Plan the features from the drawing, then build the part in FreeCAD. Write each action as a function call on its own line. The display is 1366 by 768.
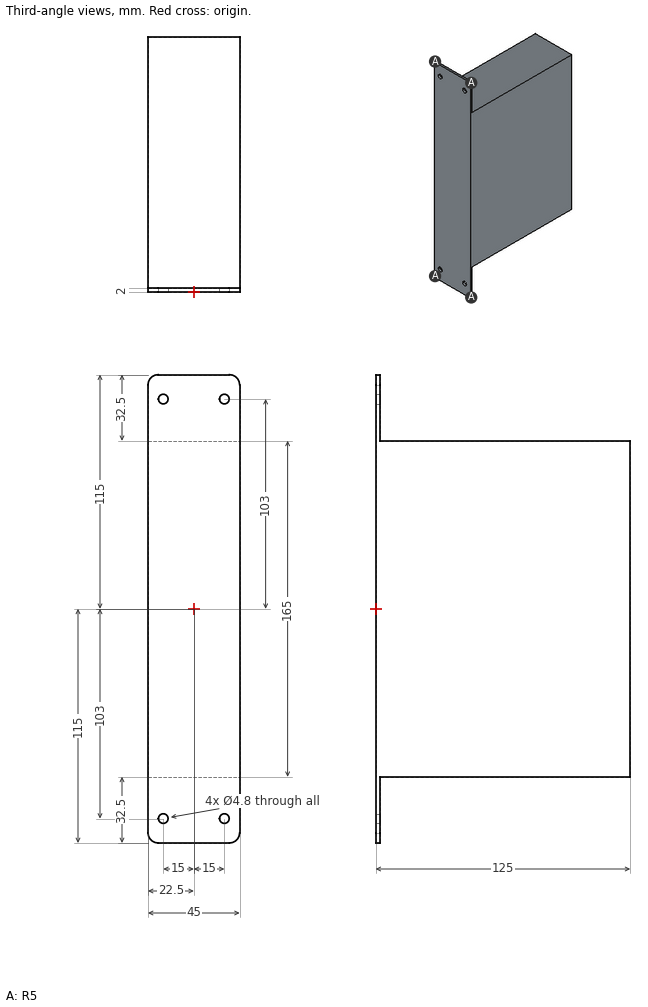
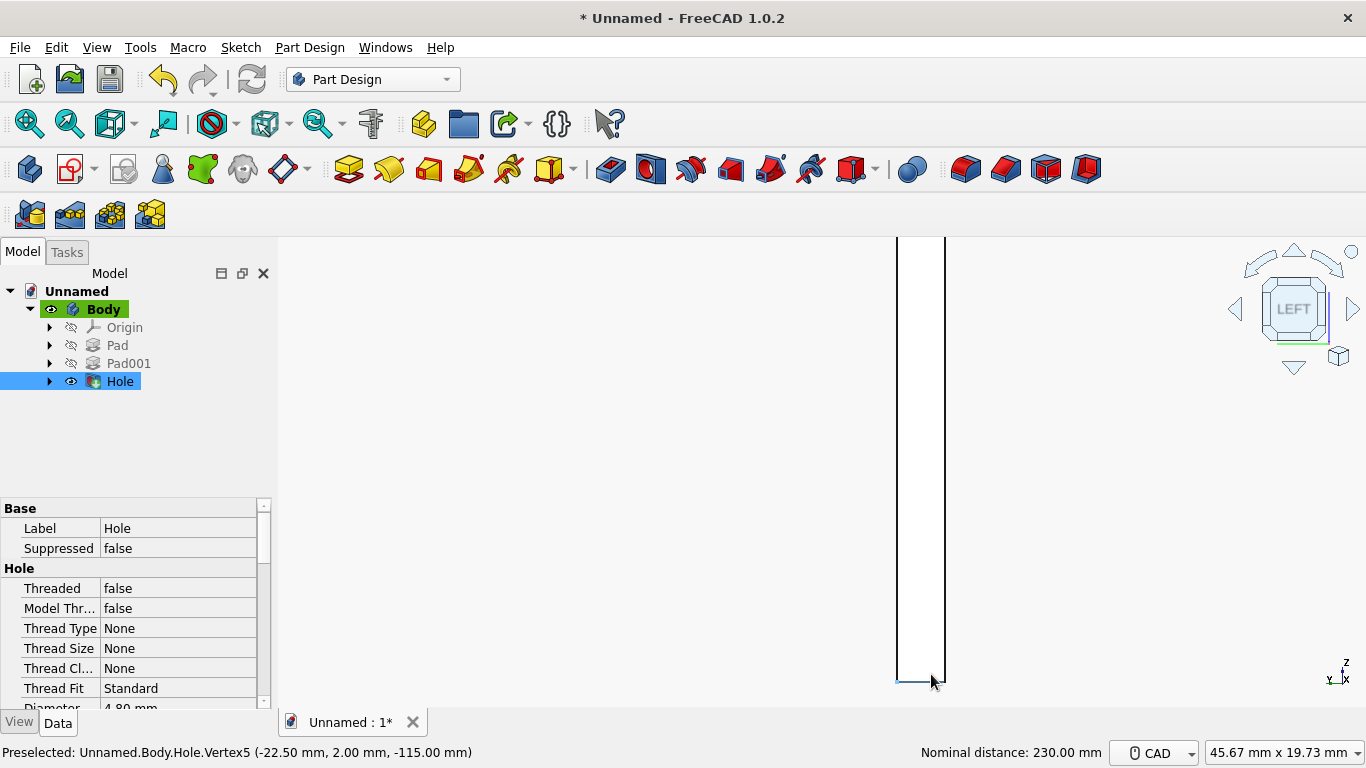
key(v)
key(f)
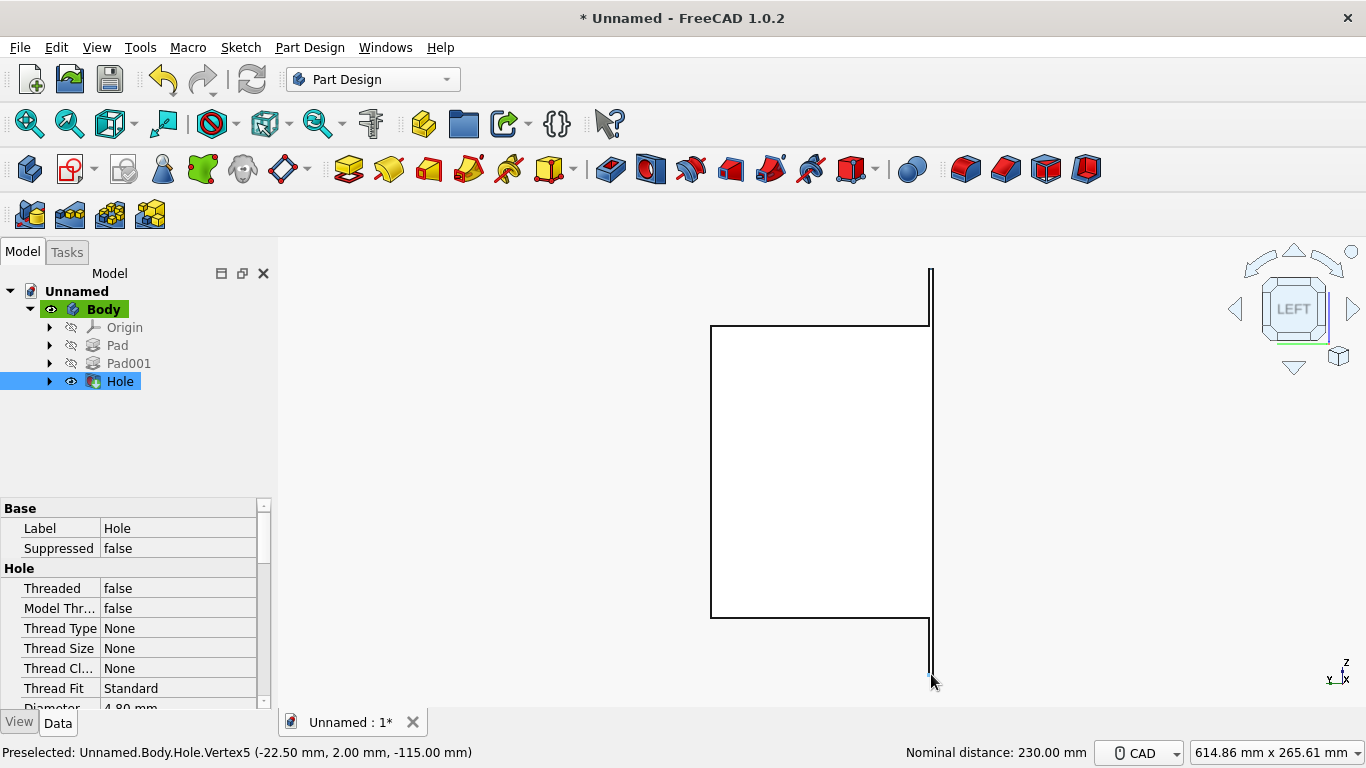
key(v)
key(3)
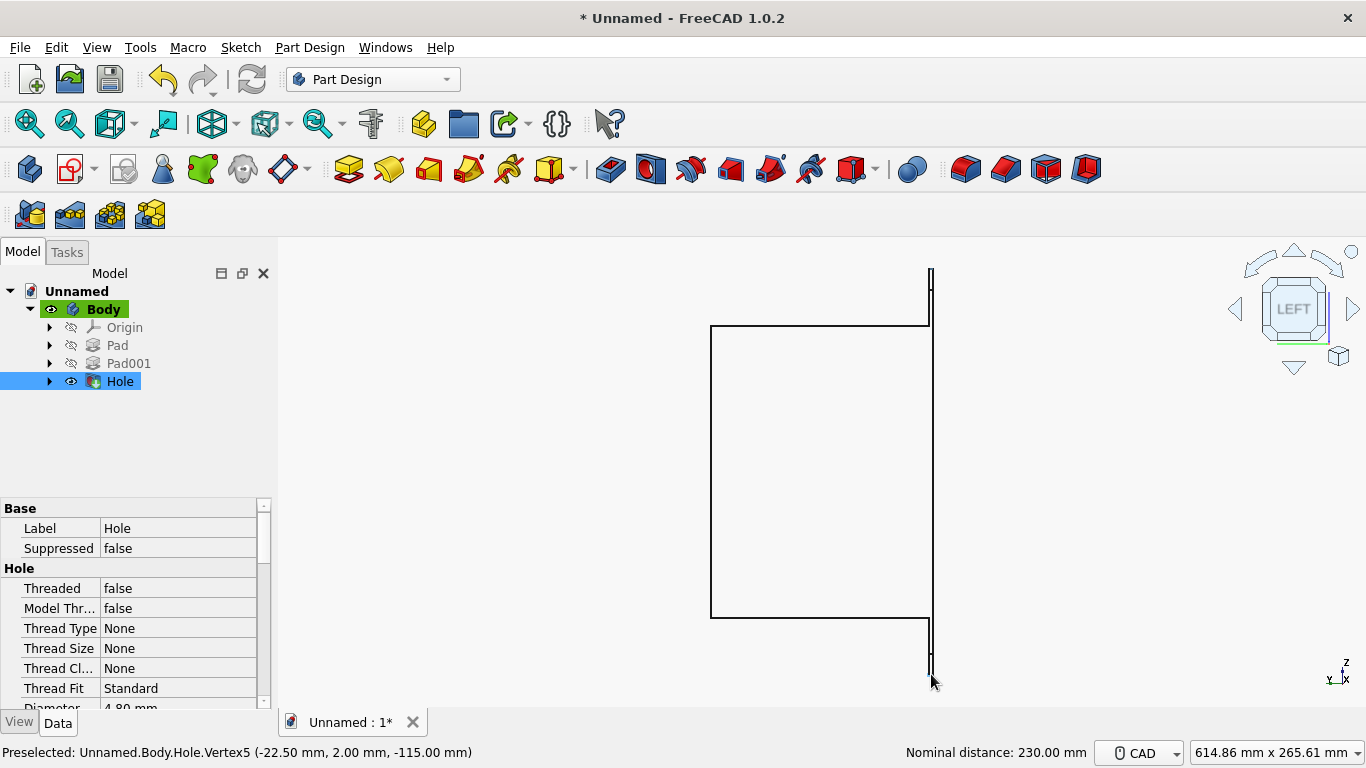
key(0)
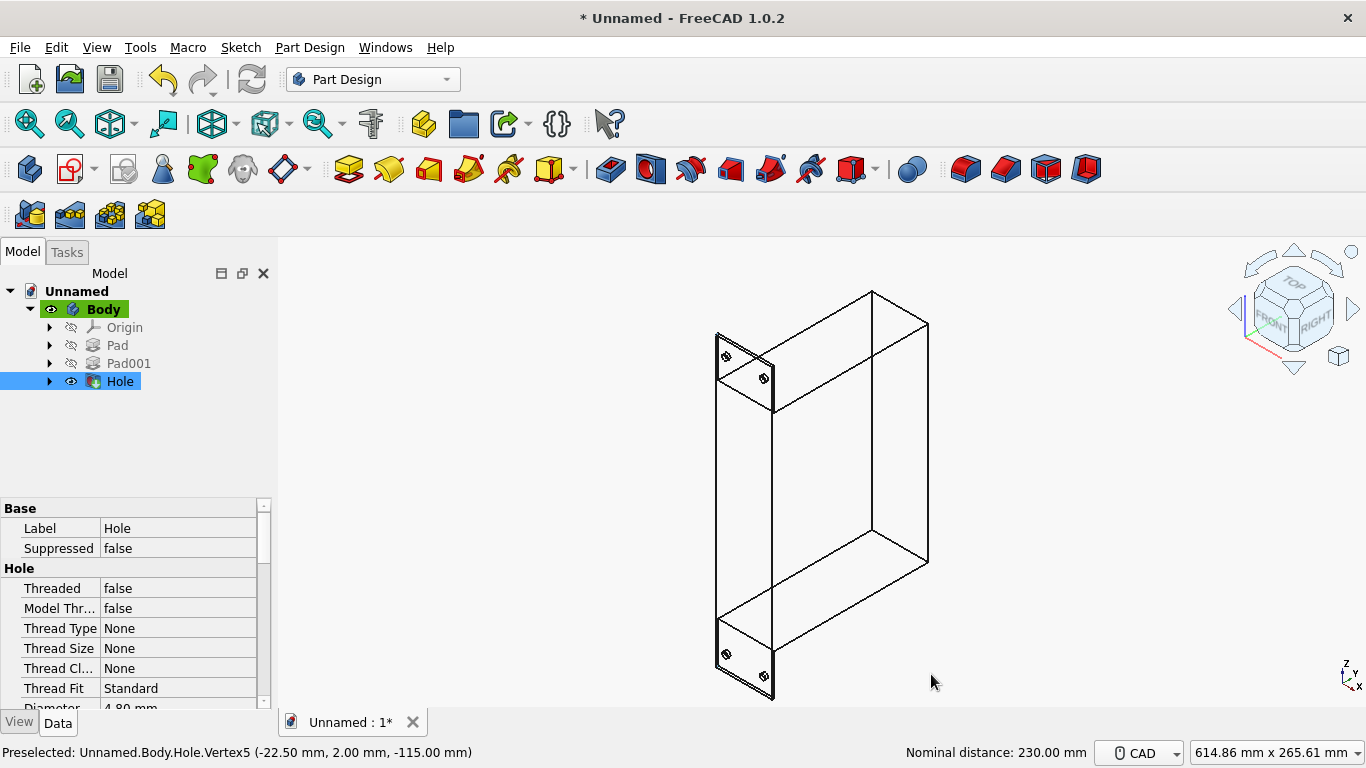
key(2)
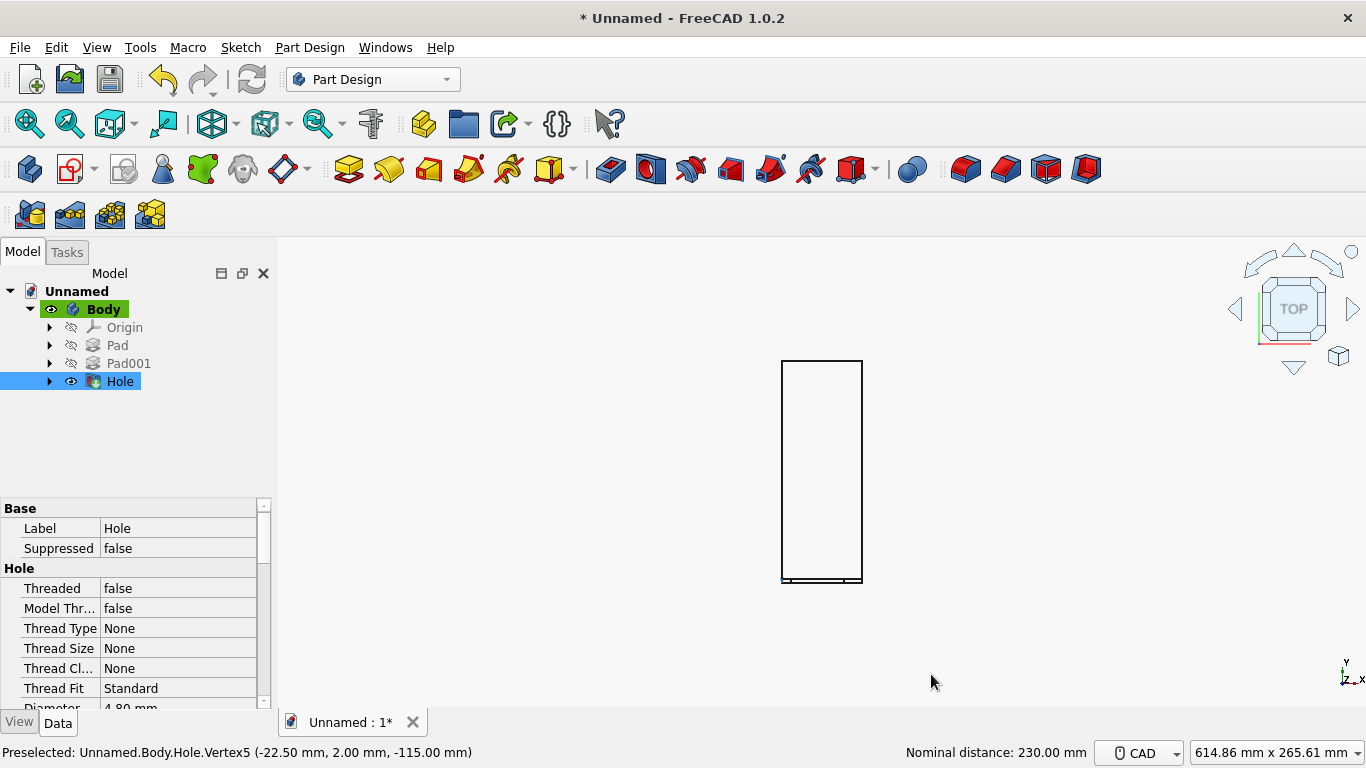
scroll(862, 580, up, 13)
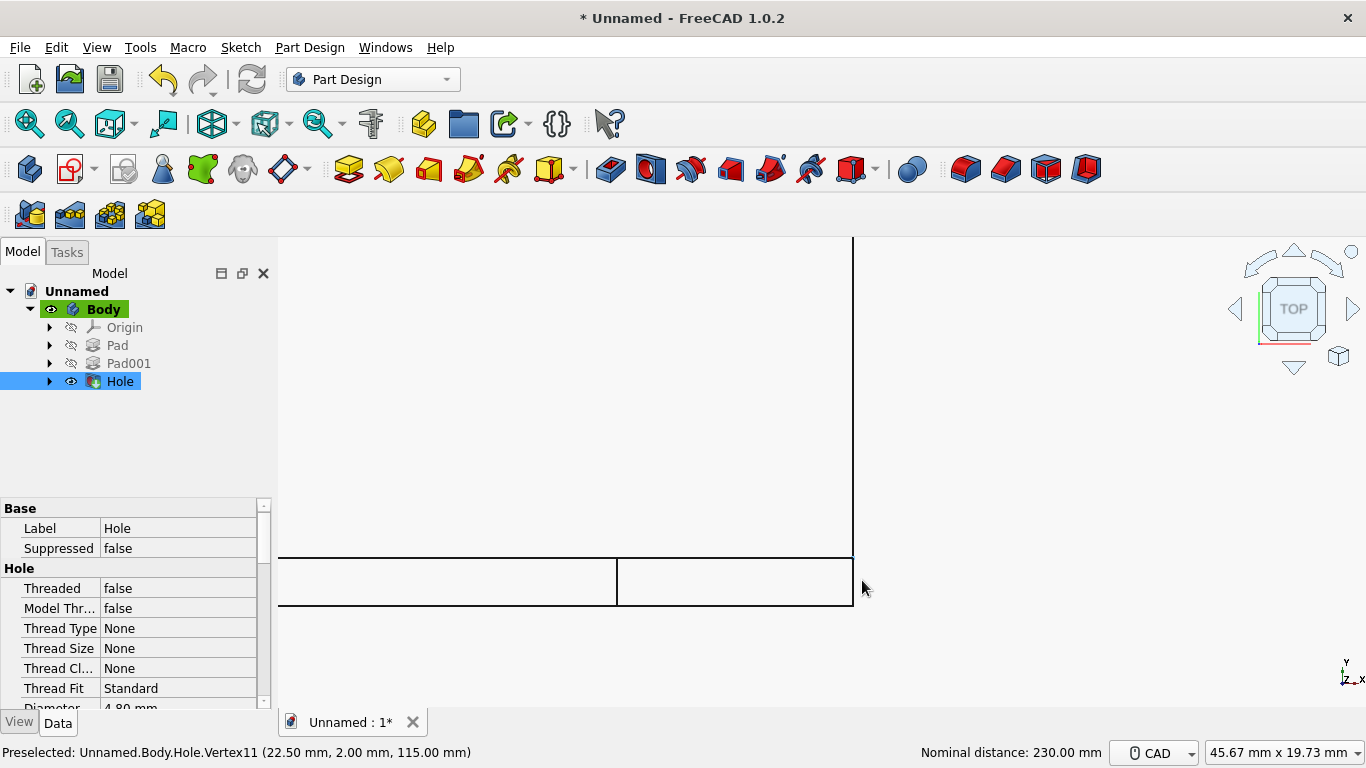
click(853, 581, ctrl)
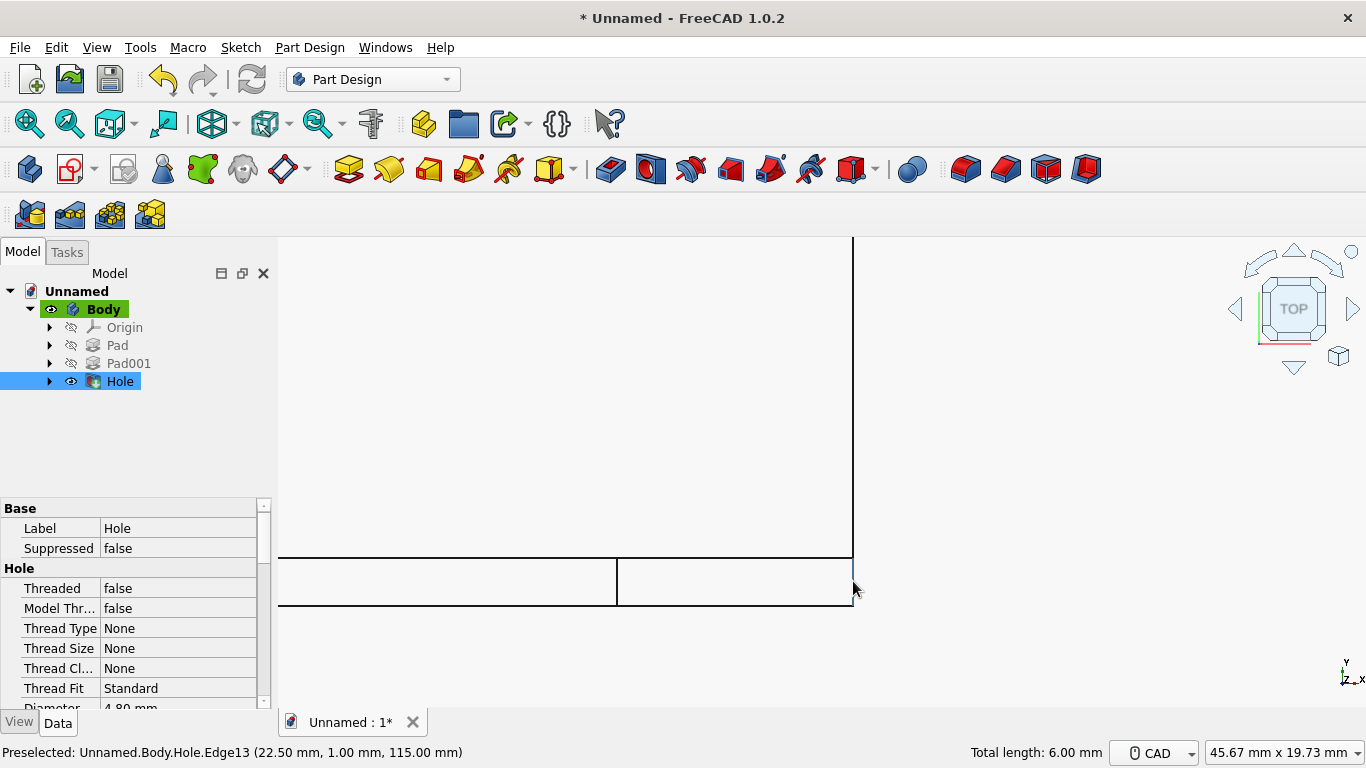
key(v)
key(f)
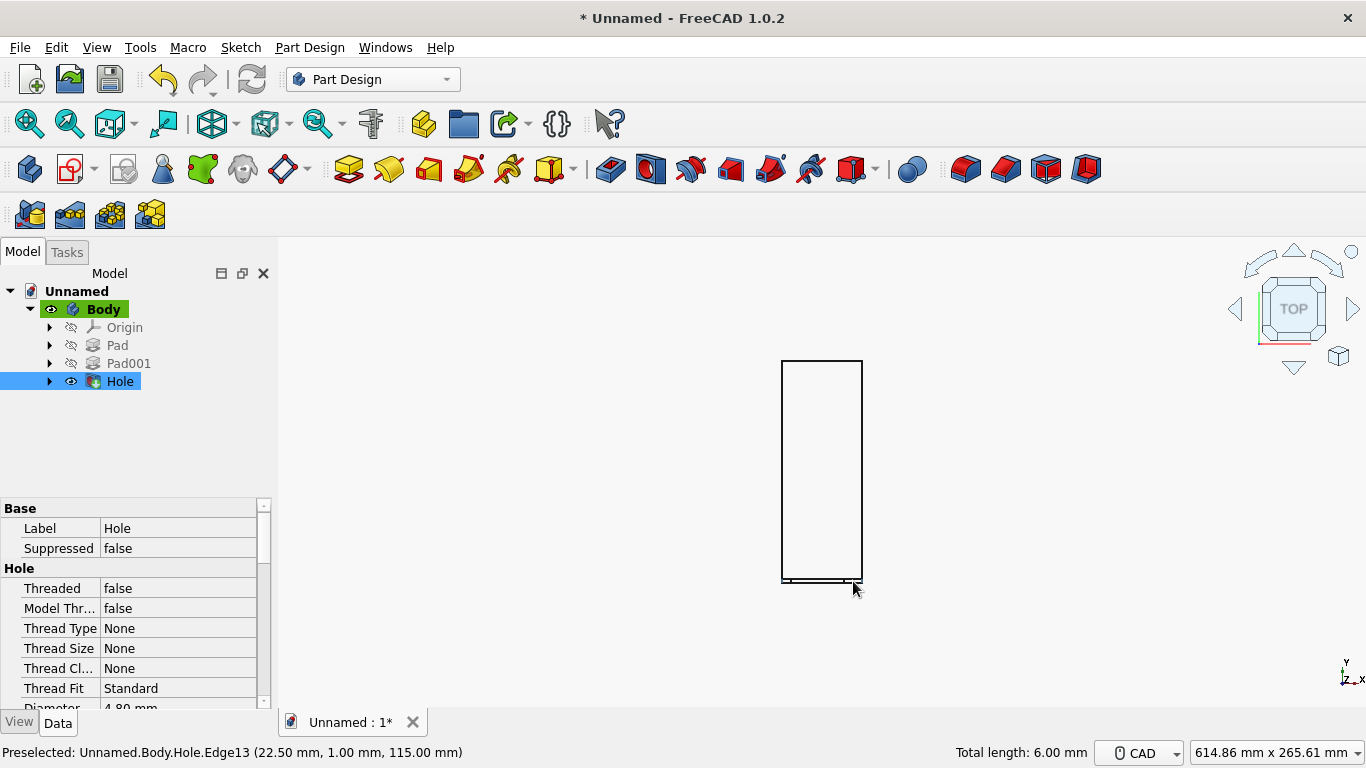
key(1)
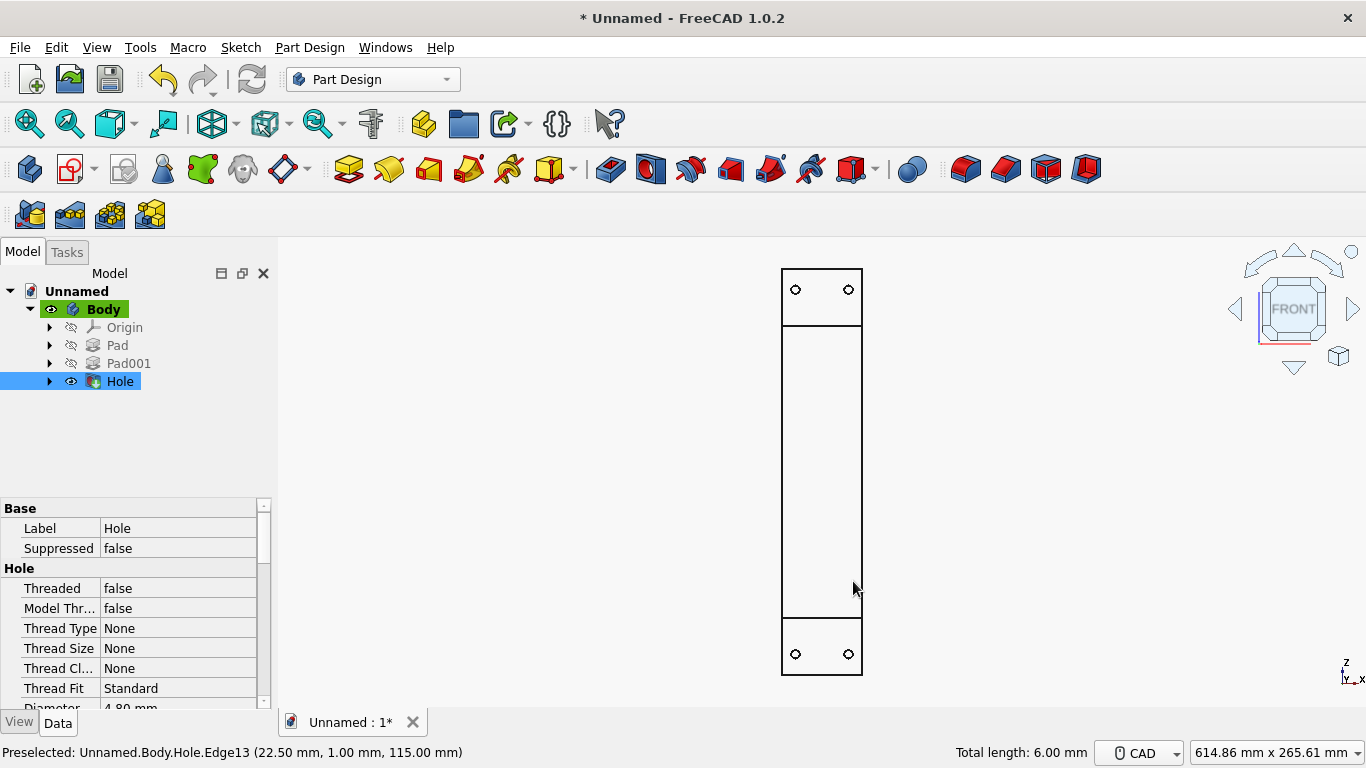
scroll(862, 674, up, 13)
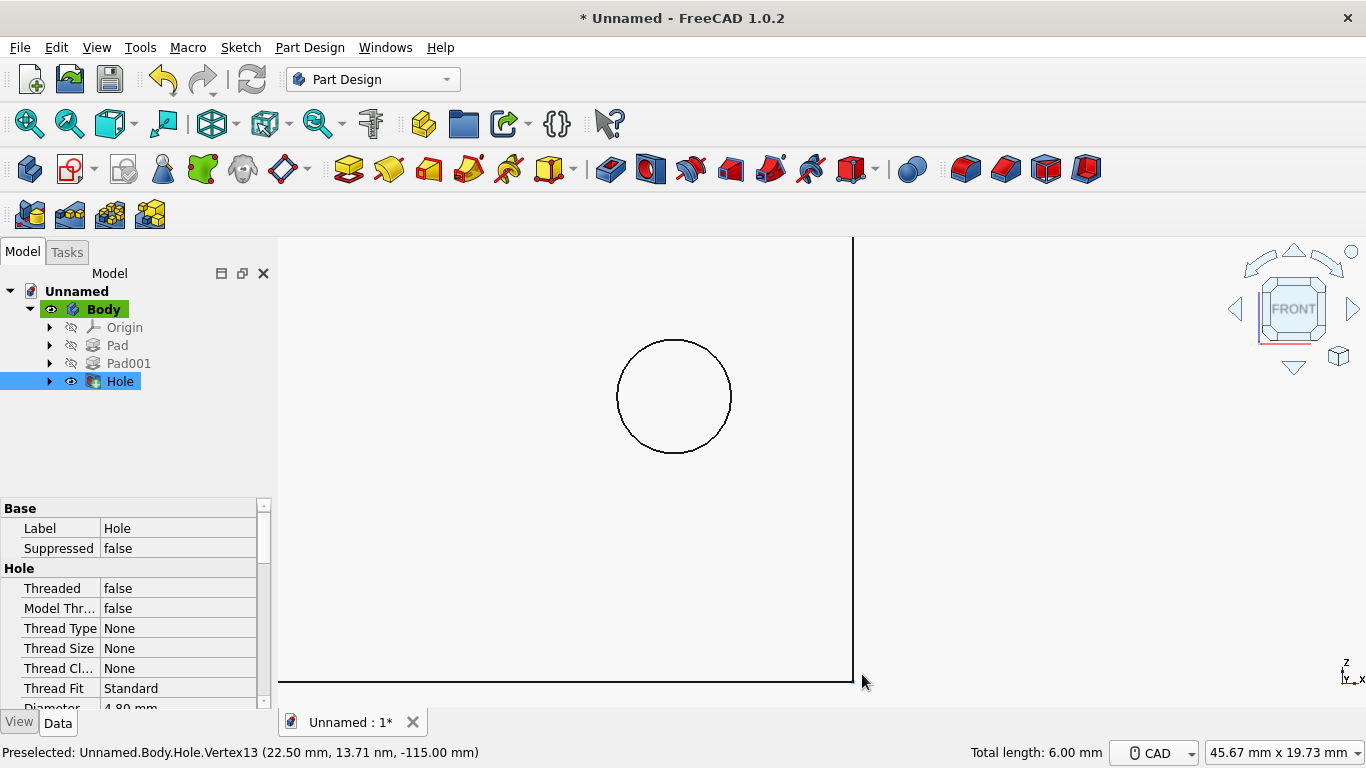
key(v)
key(f)